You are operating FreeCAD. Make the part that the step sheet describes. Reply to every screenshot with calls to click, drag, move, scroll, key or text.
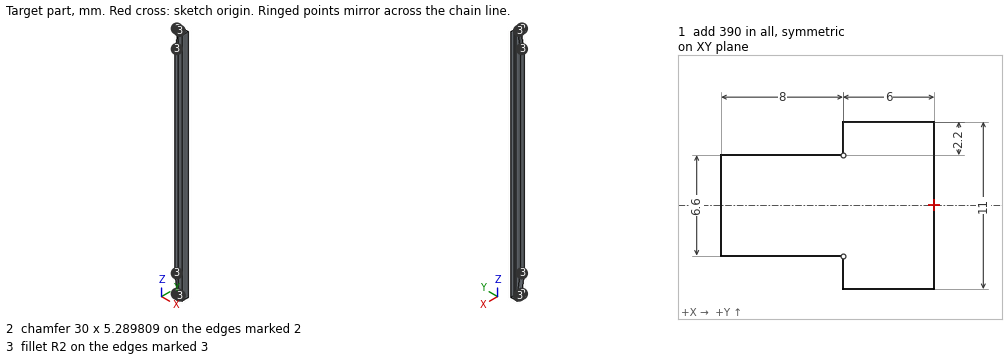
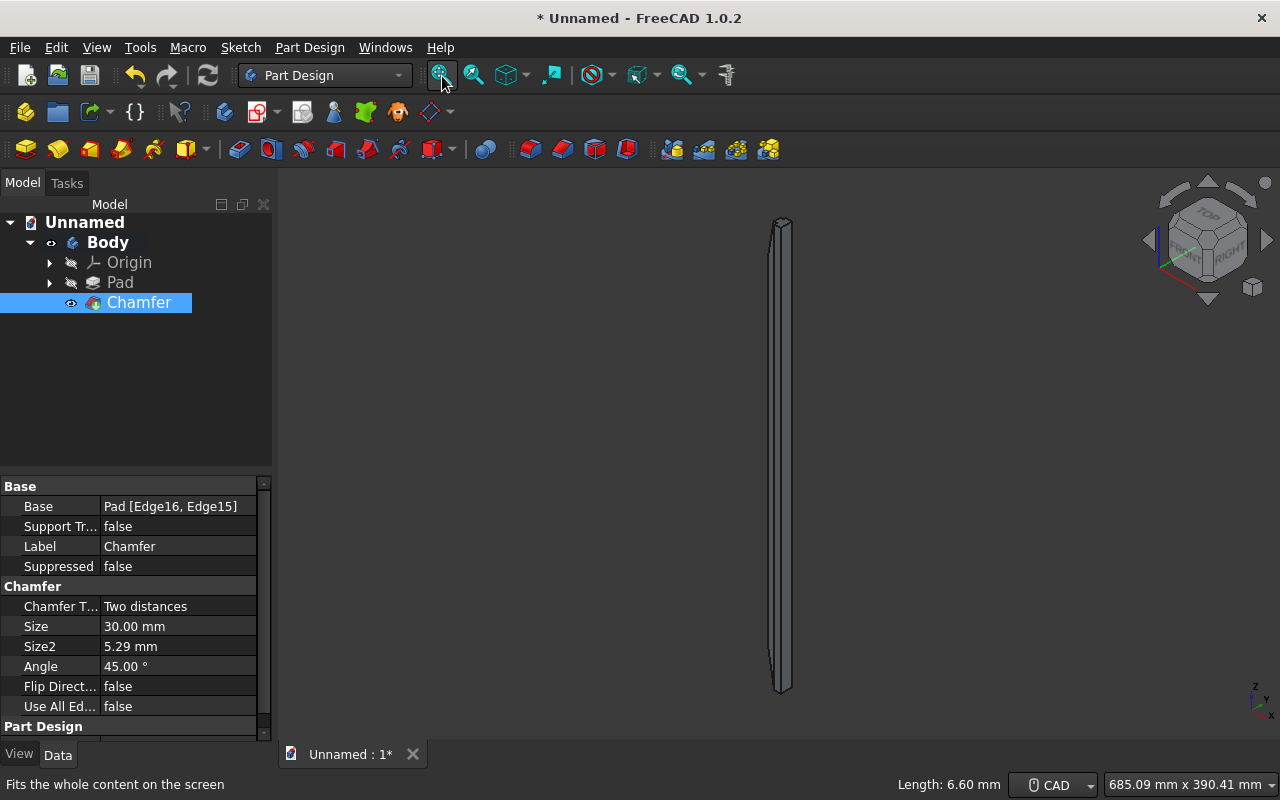
key(2)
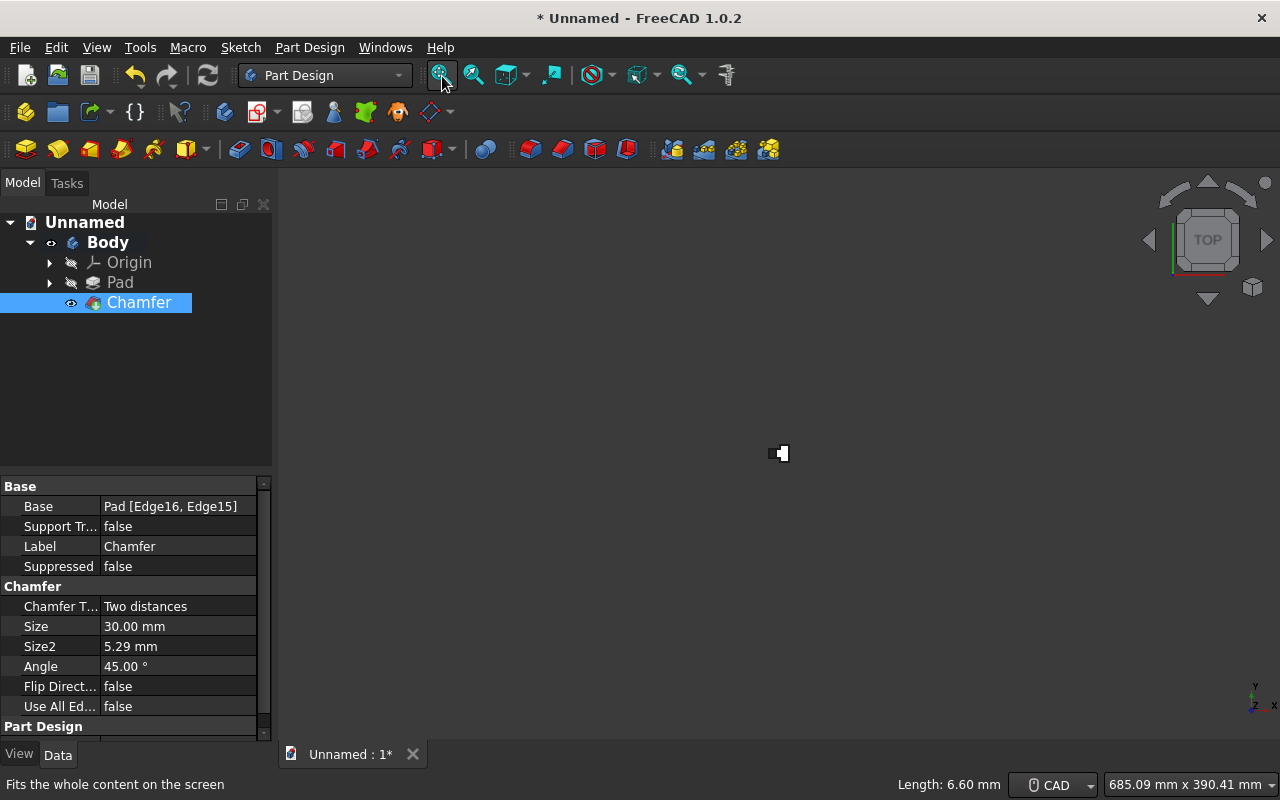
click(442, 76)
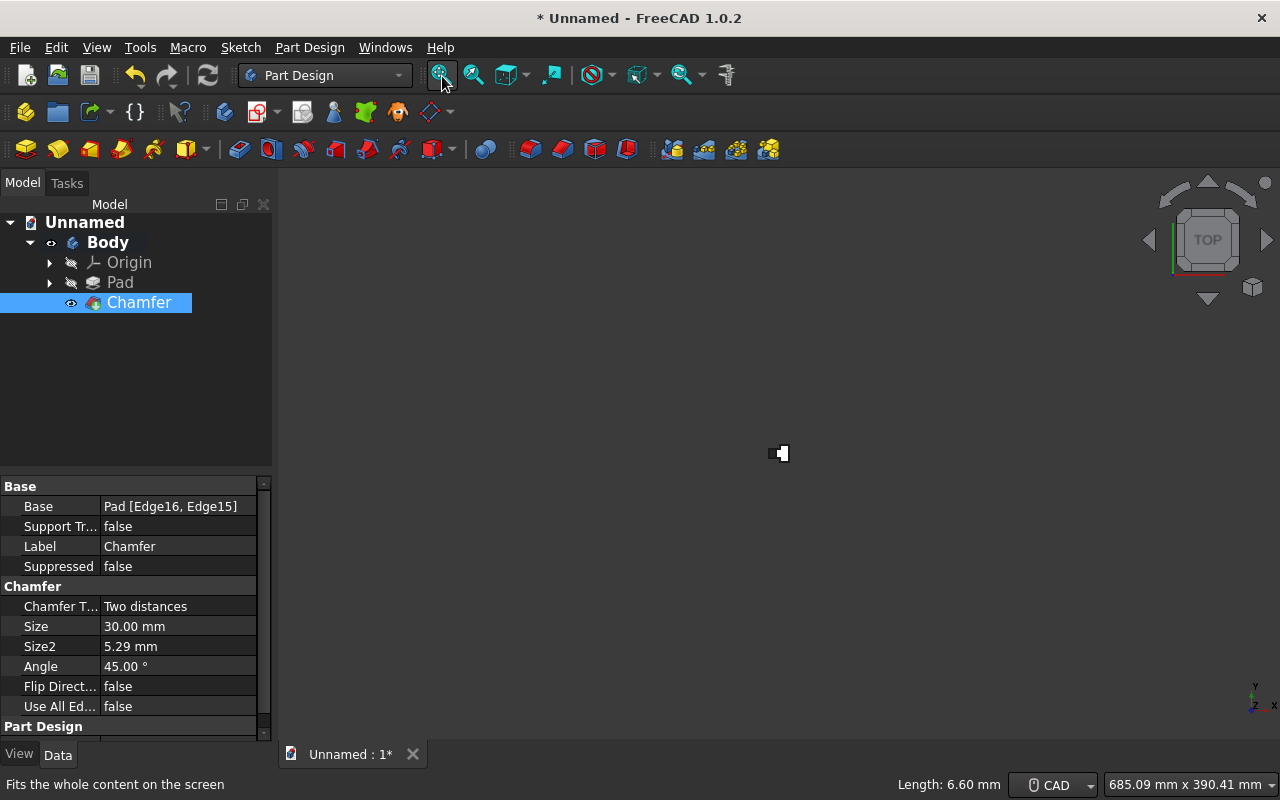
scroll(769, 452, up, 8)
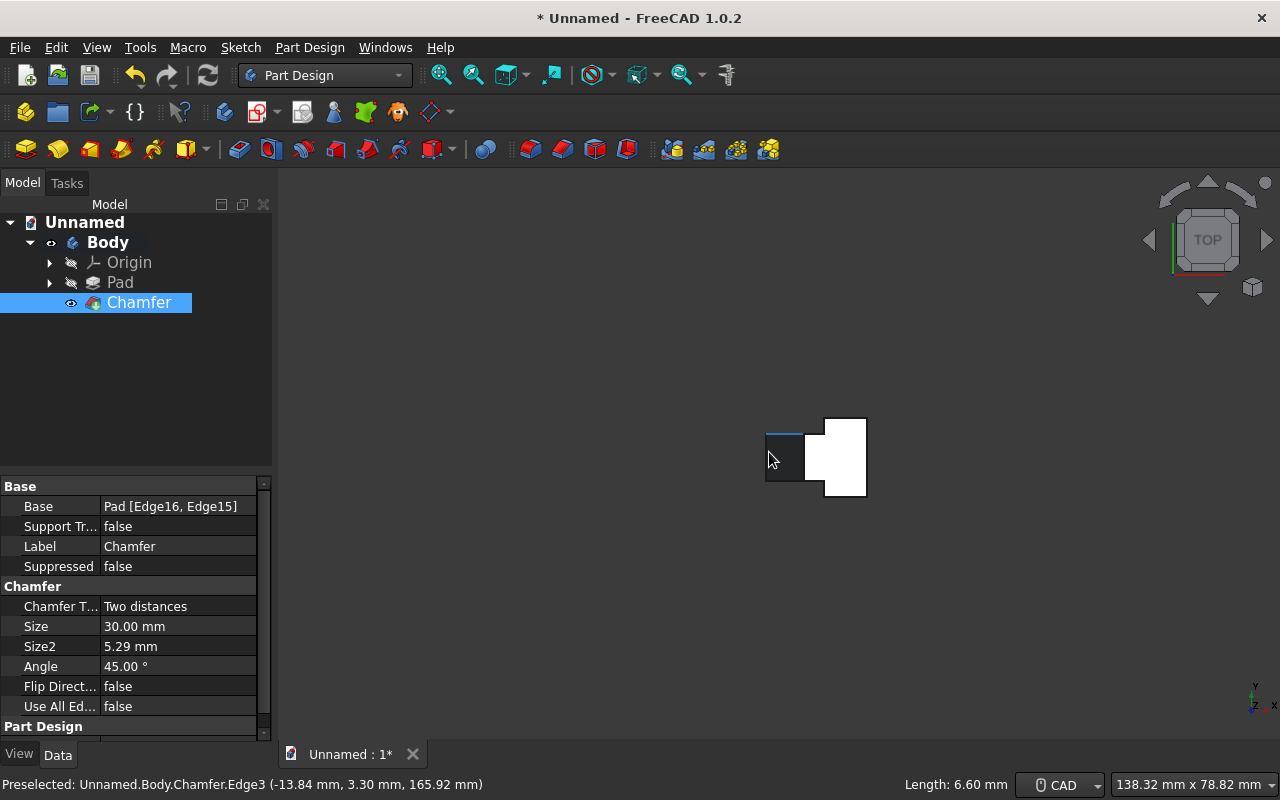
click(804, 456, ctrl)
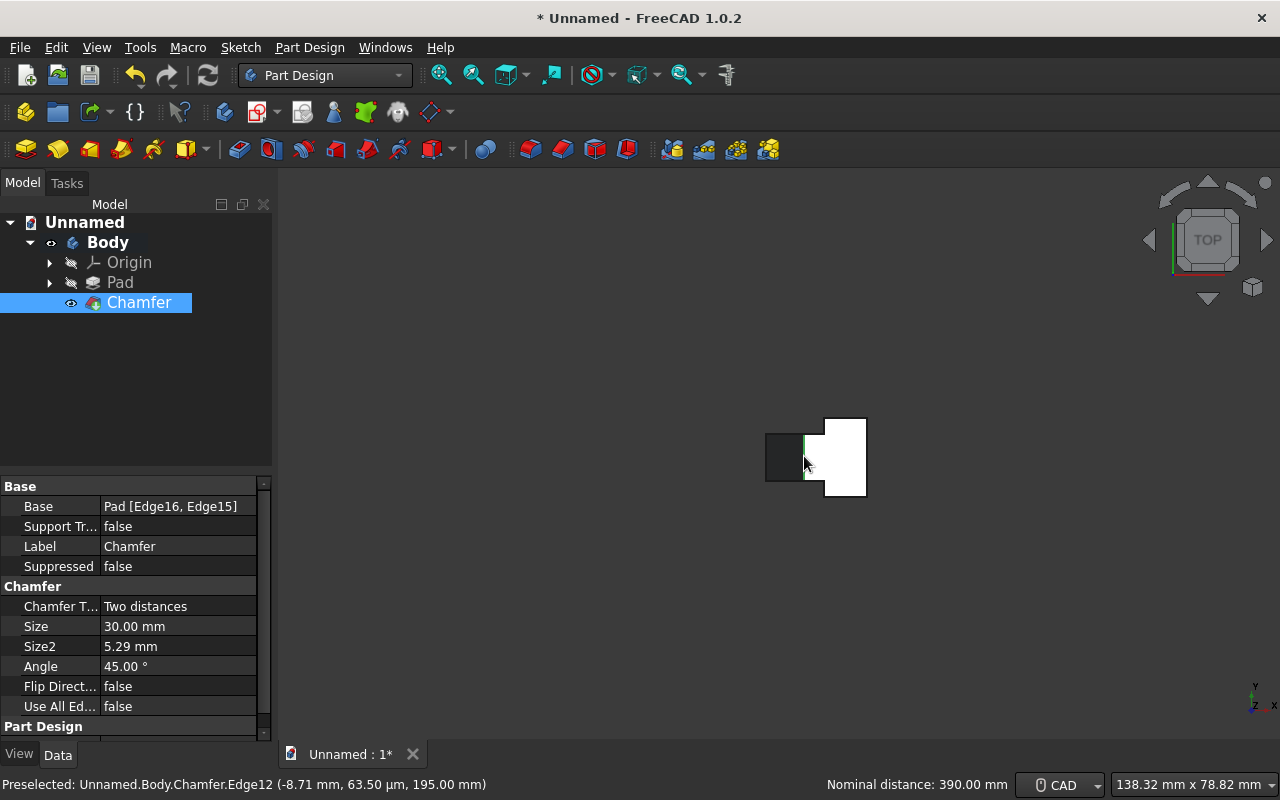
click(442, 76)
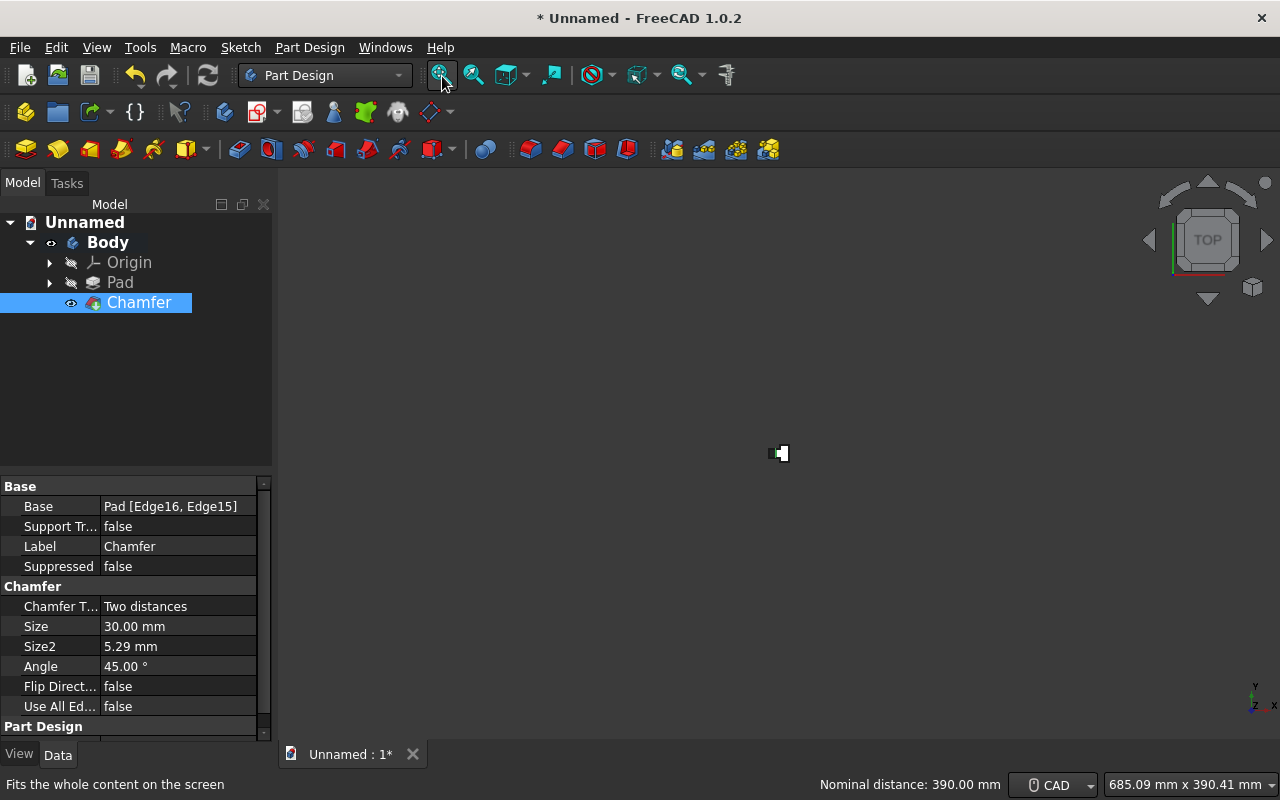
key(1)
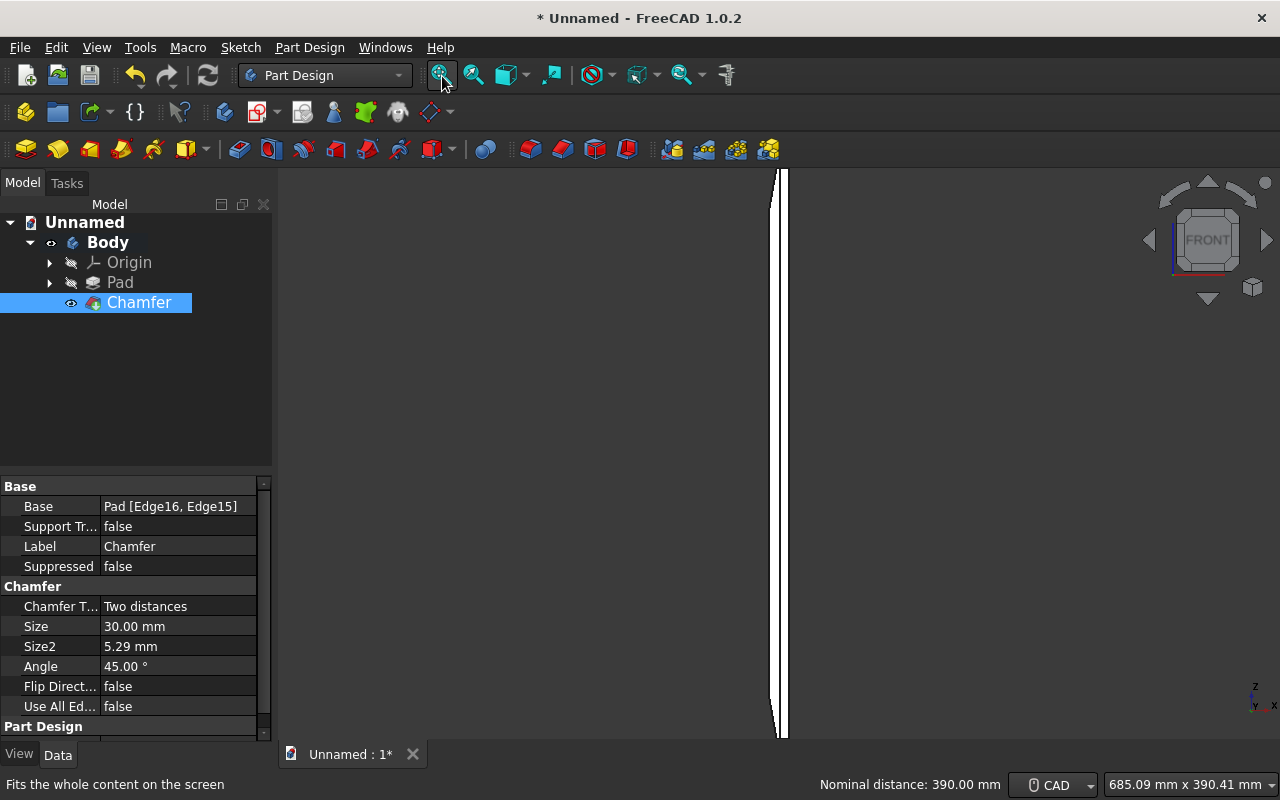
click(442, 76)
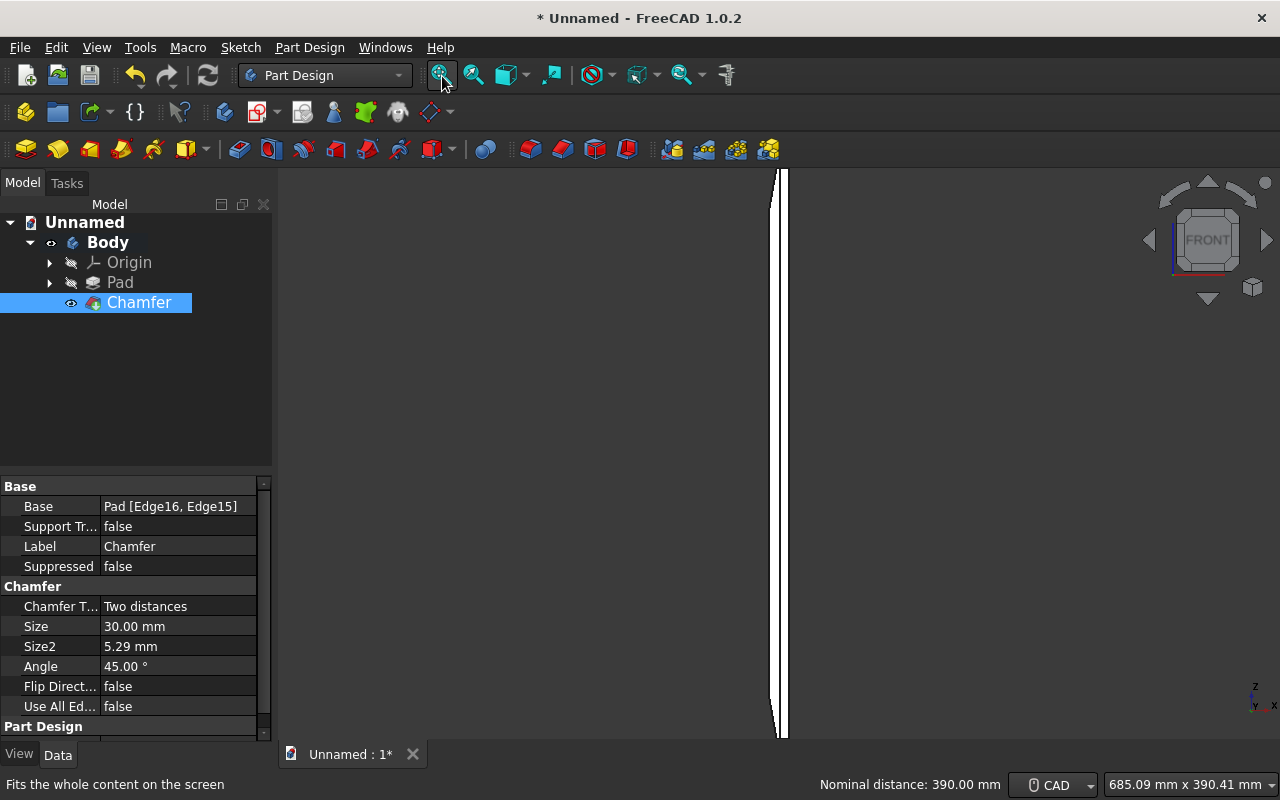
scroll(769, 211, up, 8)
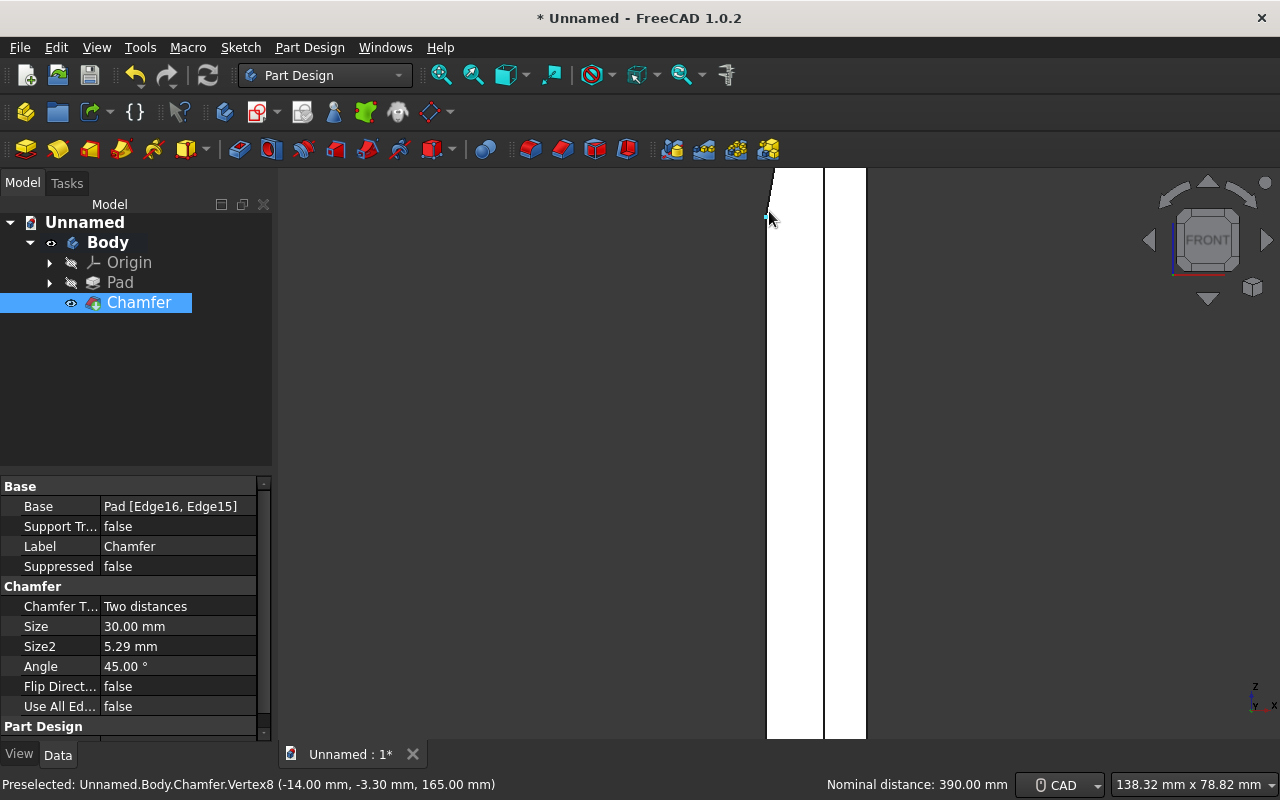
click(442, 76)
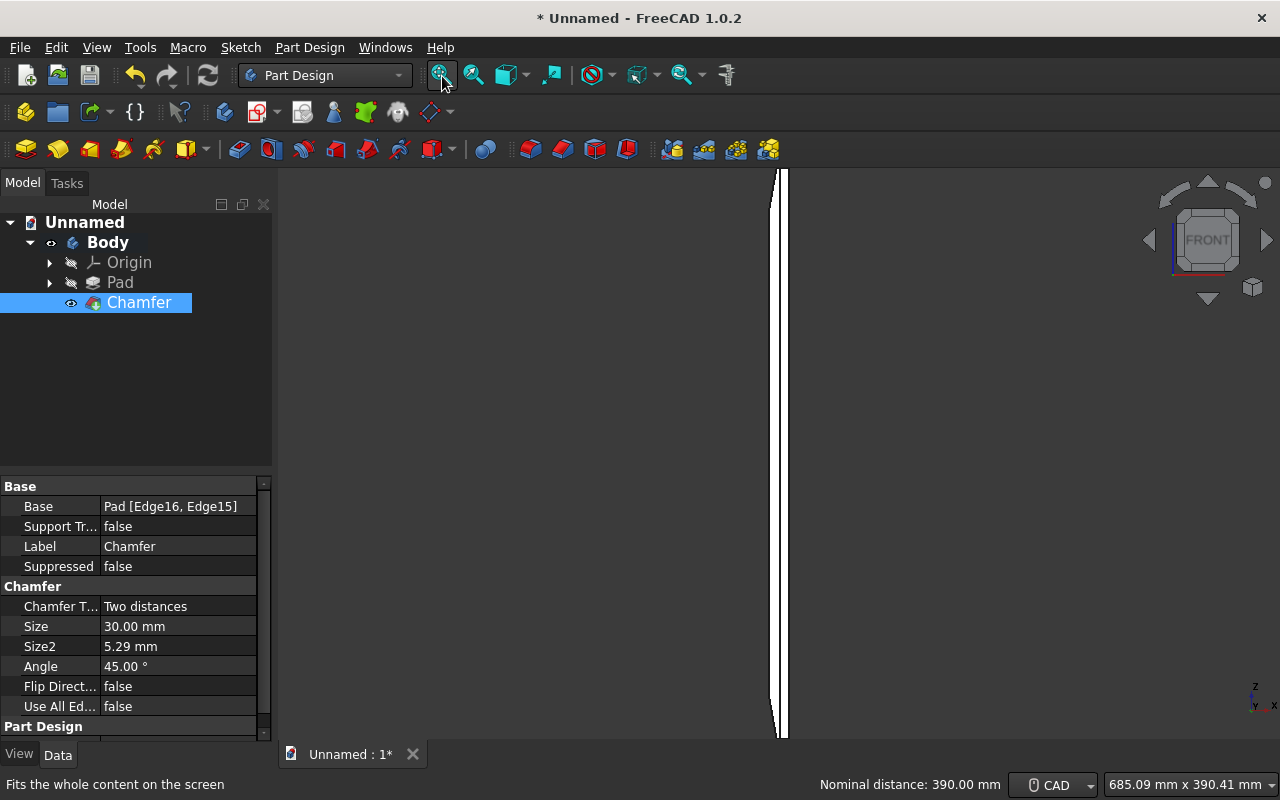
key(3)